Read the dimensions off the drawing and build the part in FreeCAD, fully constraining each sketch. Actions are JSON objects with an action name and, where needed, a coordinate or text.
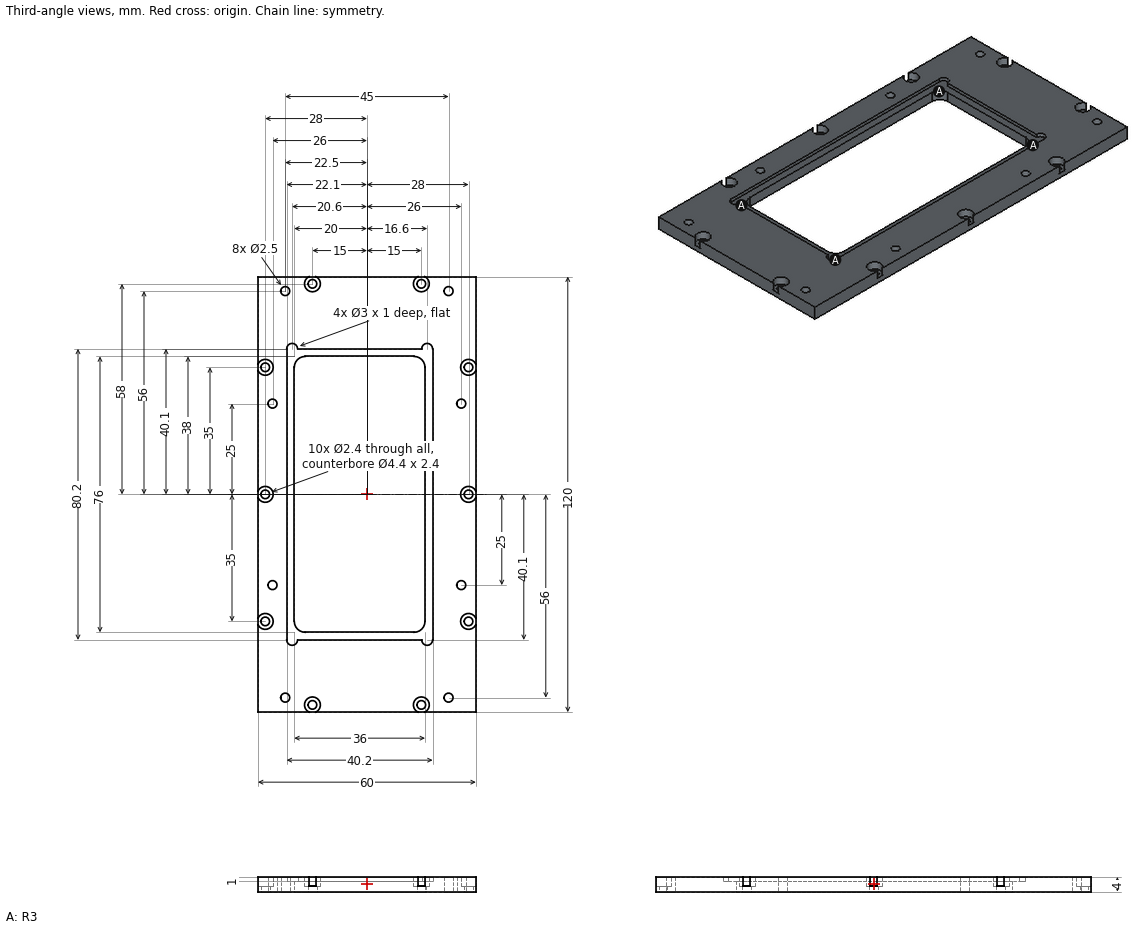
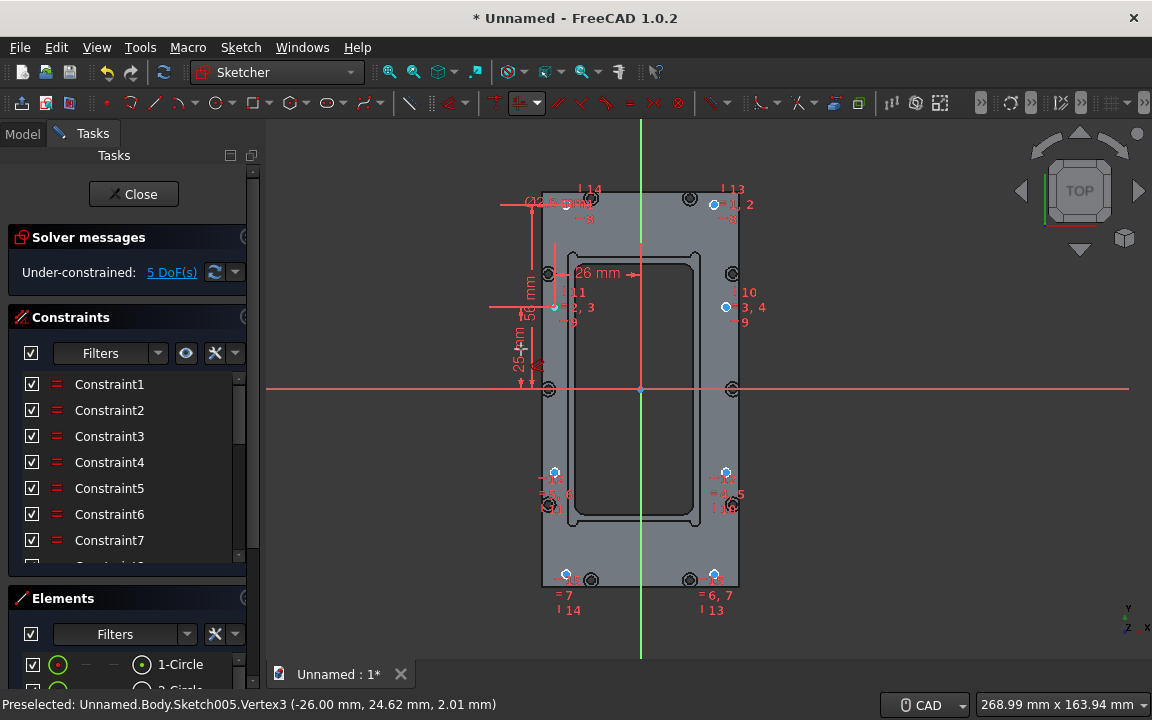
{"action": "left_click", "coordinate": [726, 307]}
{"action": "left_click", "coordinate": [683, 273]}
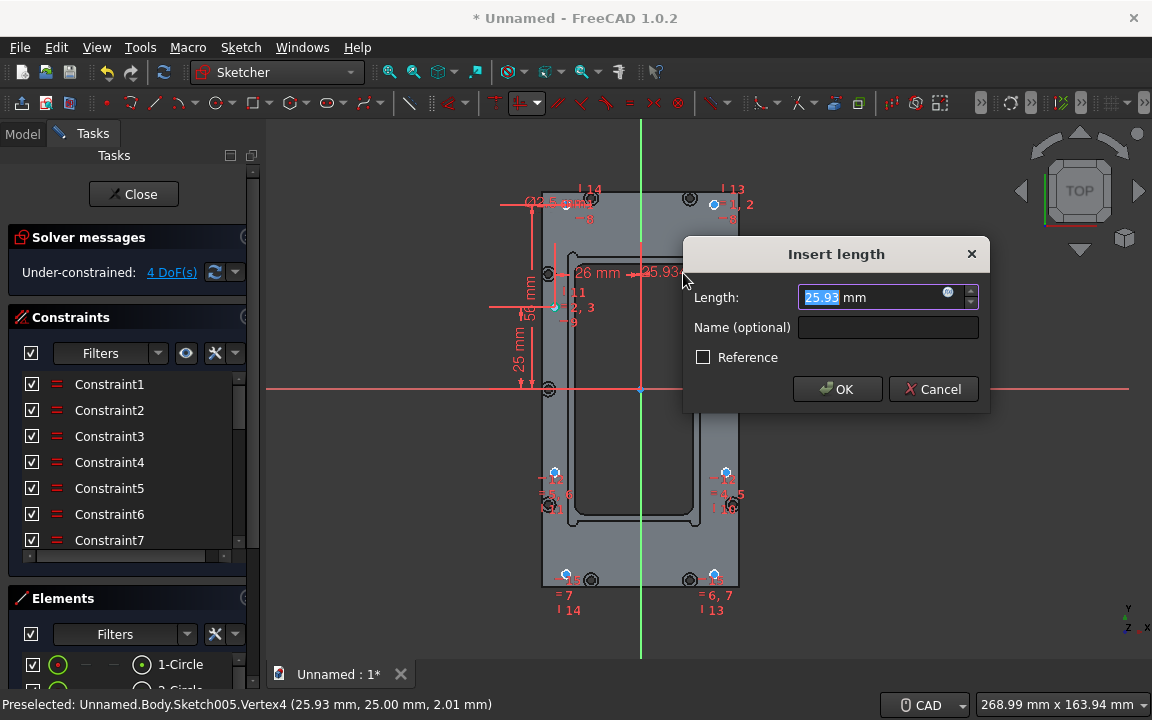
{"action": "type", "text": "26"}
{"action": "key", "text": "Return"}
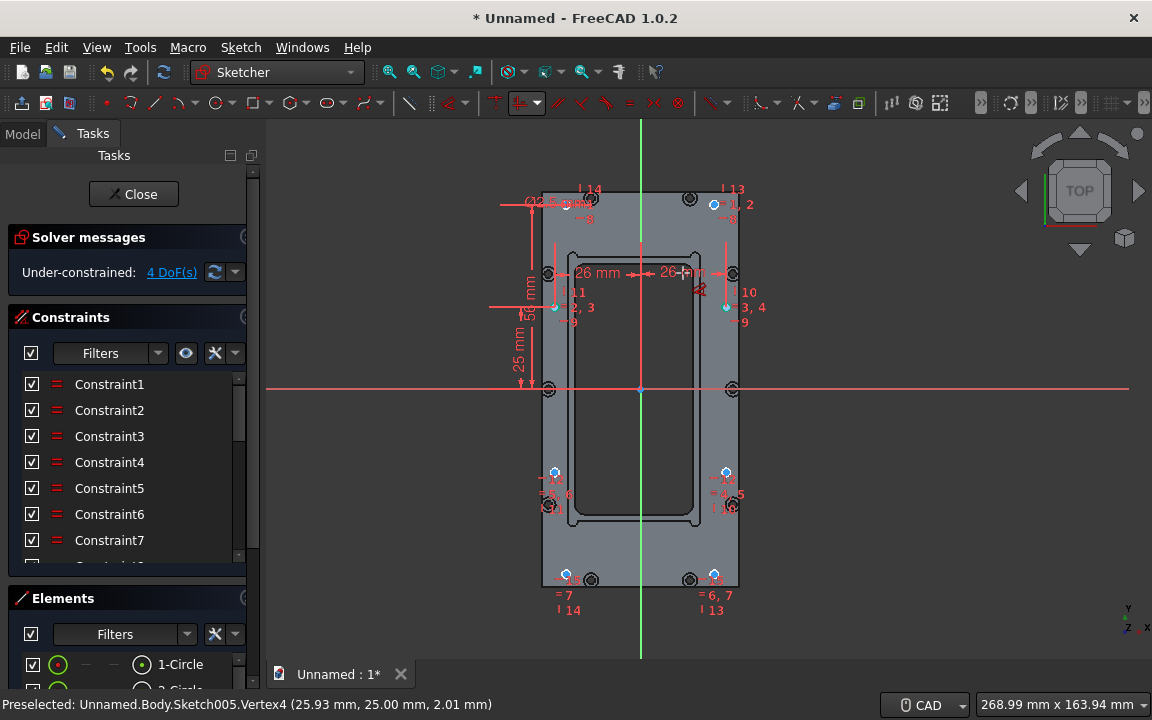
{"action": "left_click", "coordinate": [726, 472]}
{"action": "left_click", "coordinate": [760, 431]}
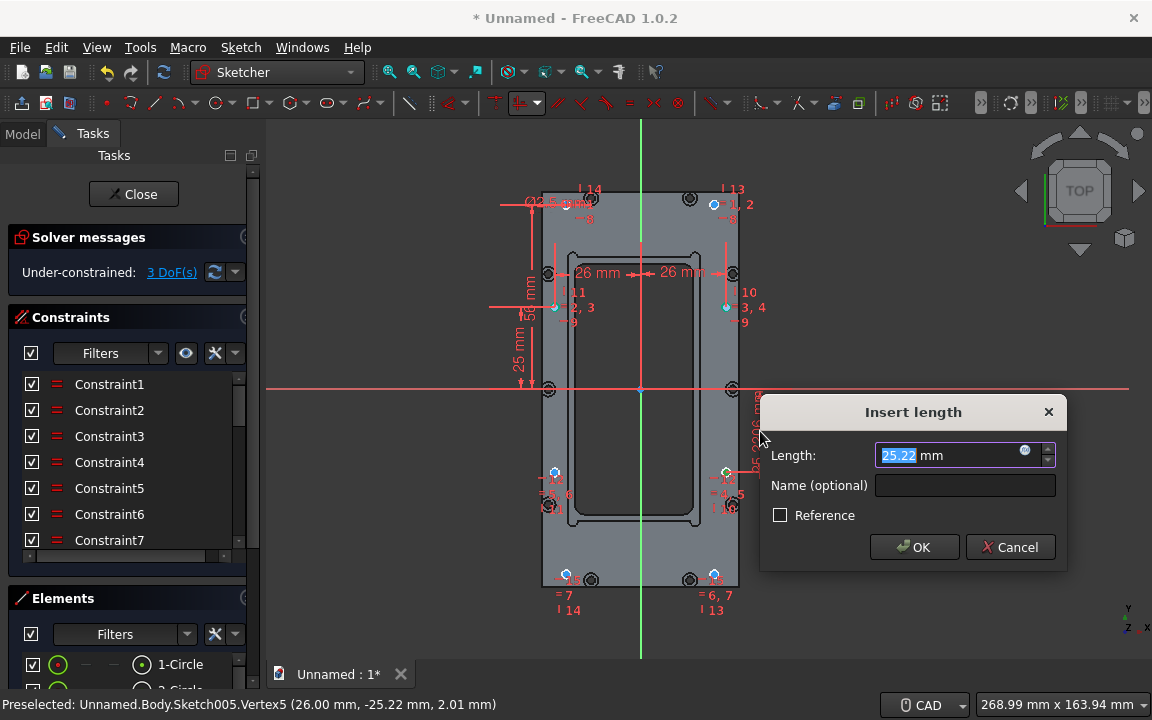
{"action": "type", "text": "25"}
{"action": "key", "text": "Return"}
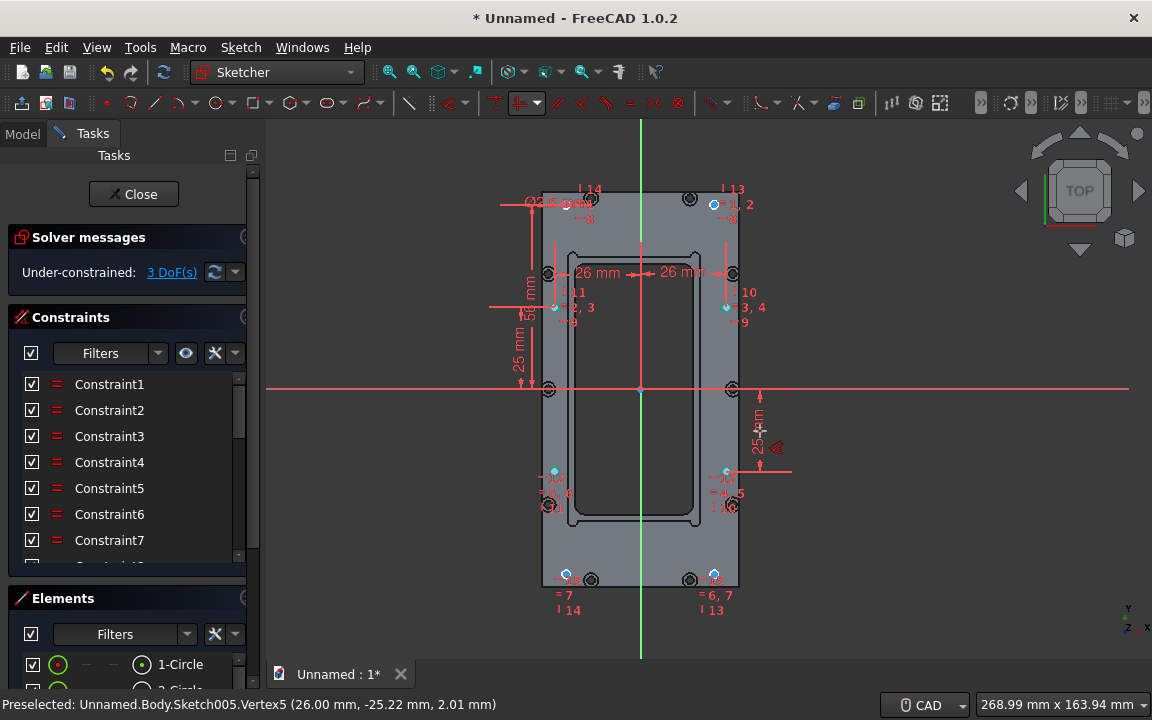
{"action": "left_click", "coordinate": [714, 574]}
{"action": "left_click", "coordinate": [748, 482]}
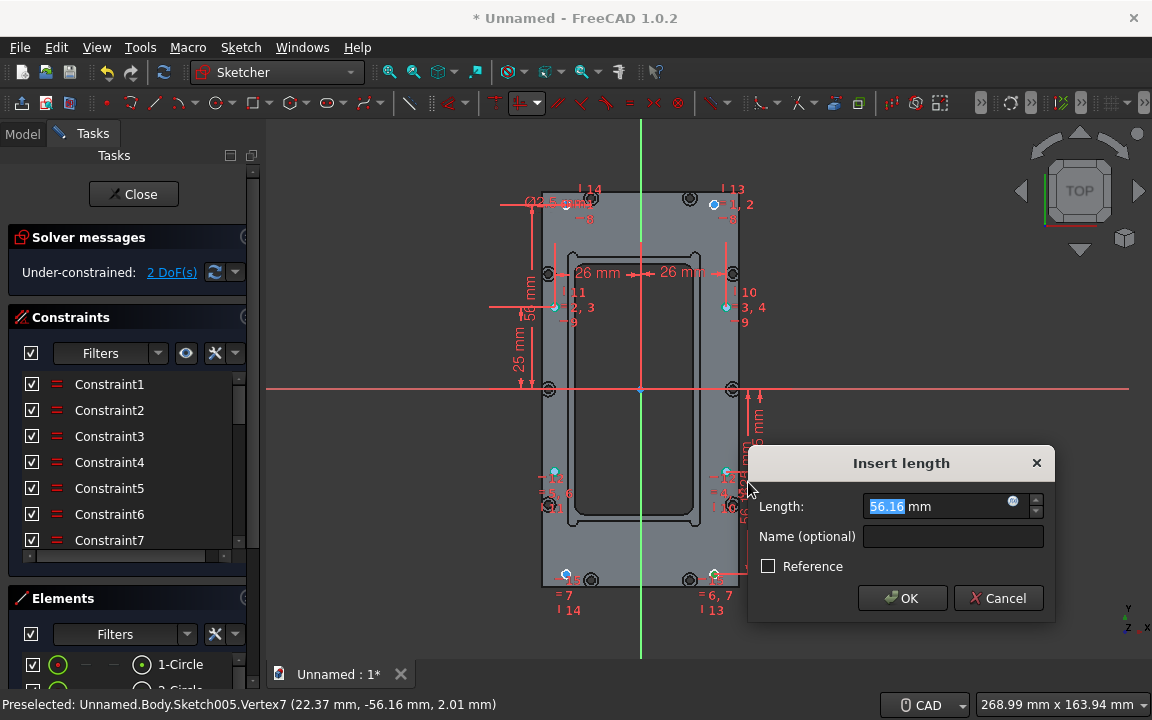
{"action": "type", "text": "56"}
{"action": "key", "text": "Return"}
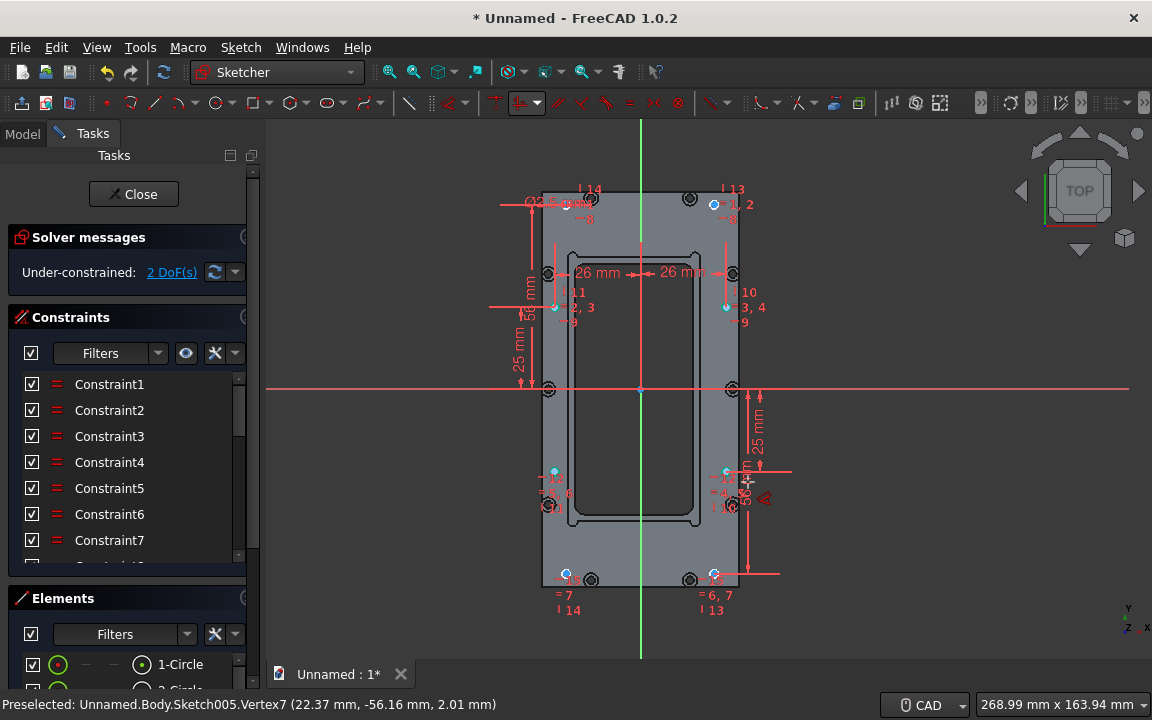
{"action": "left_click", "coordinate": [566, 205]}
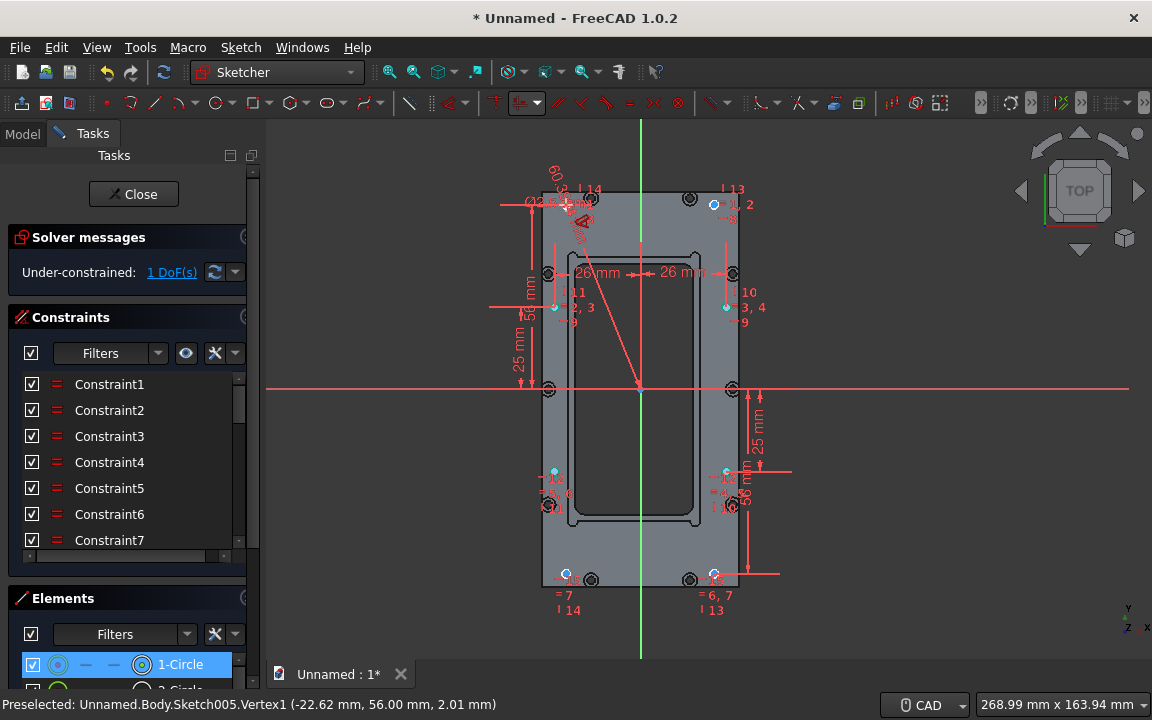
{"action": "left_click", "coordinate": [714, 205]}
{"action": "left_click", "coordinate": [606, 171]}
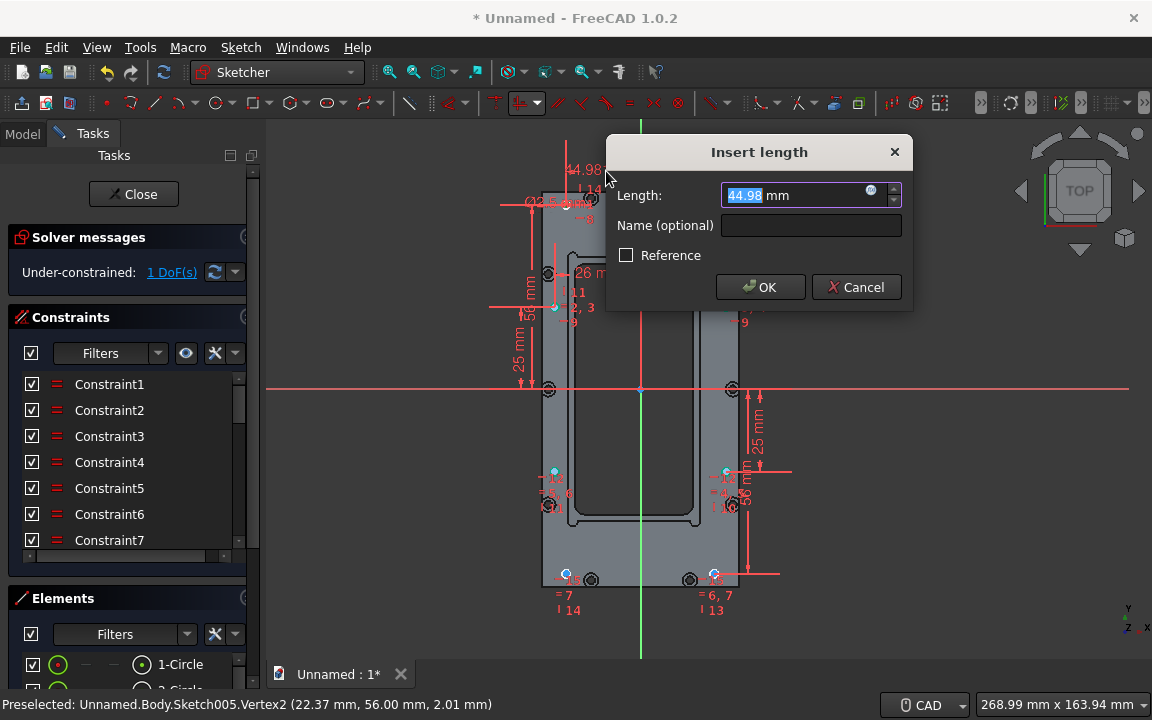
{"action": "type", "text": "45"}
{"action": "key", "text": "Return"}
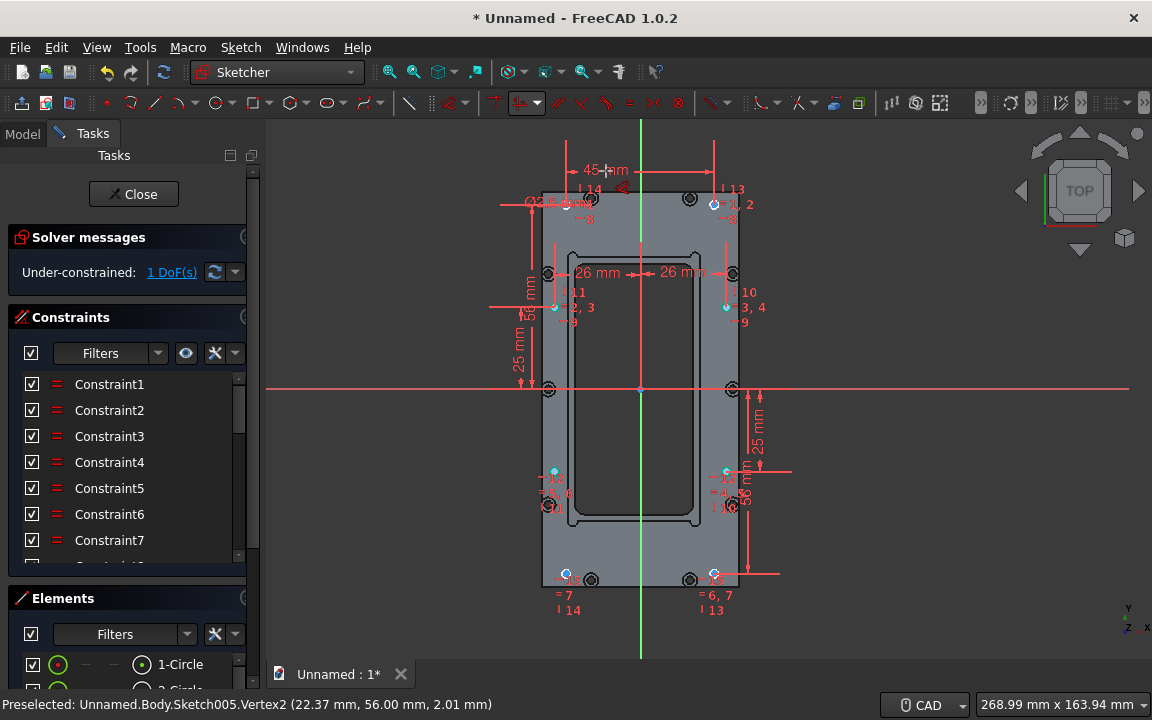
{"action": "left_click", "coordinate": [566, 205]}
{"action": "left_click", "coordinate": [603, 423]}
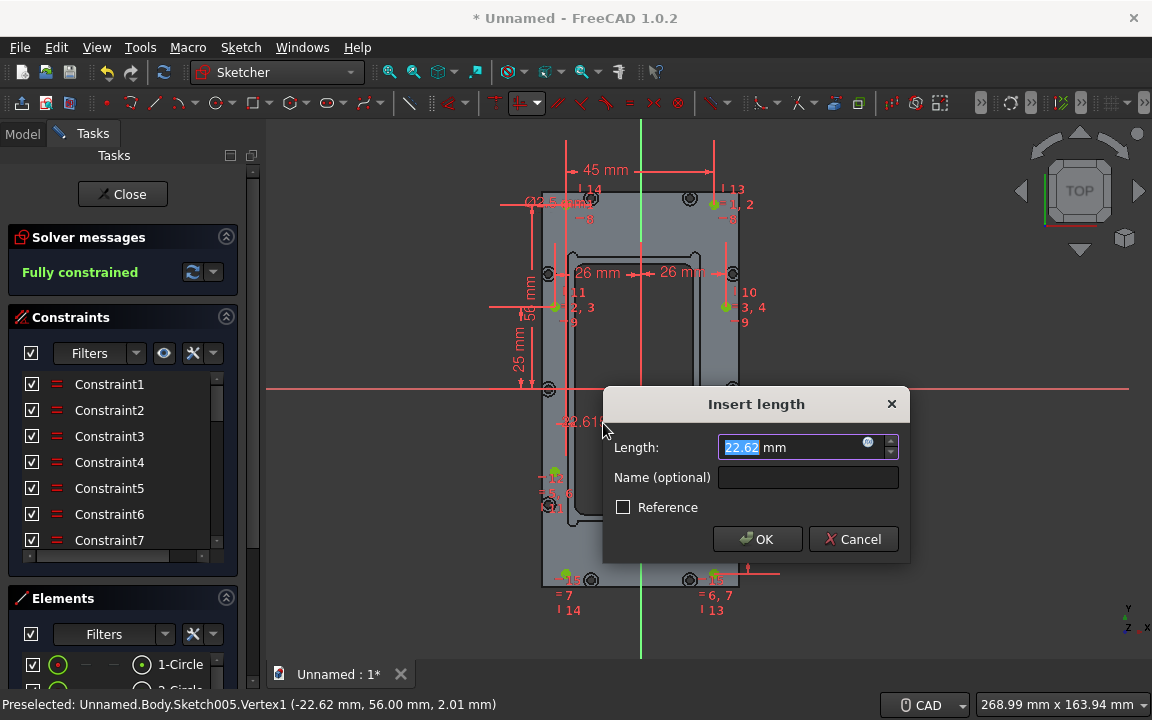
{"action": "type", "text": "22.5"}
{"action": "key", "text": "Return"}
{"action": "key", "text": "Escape"}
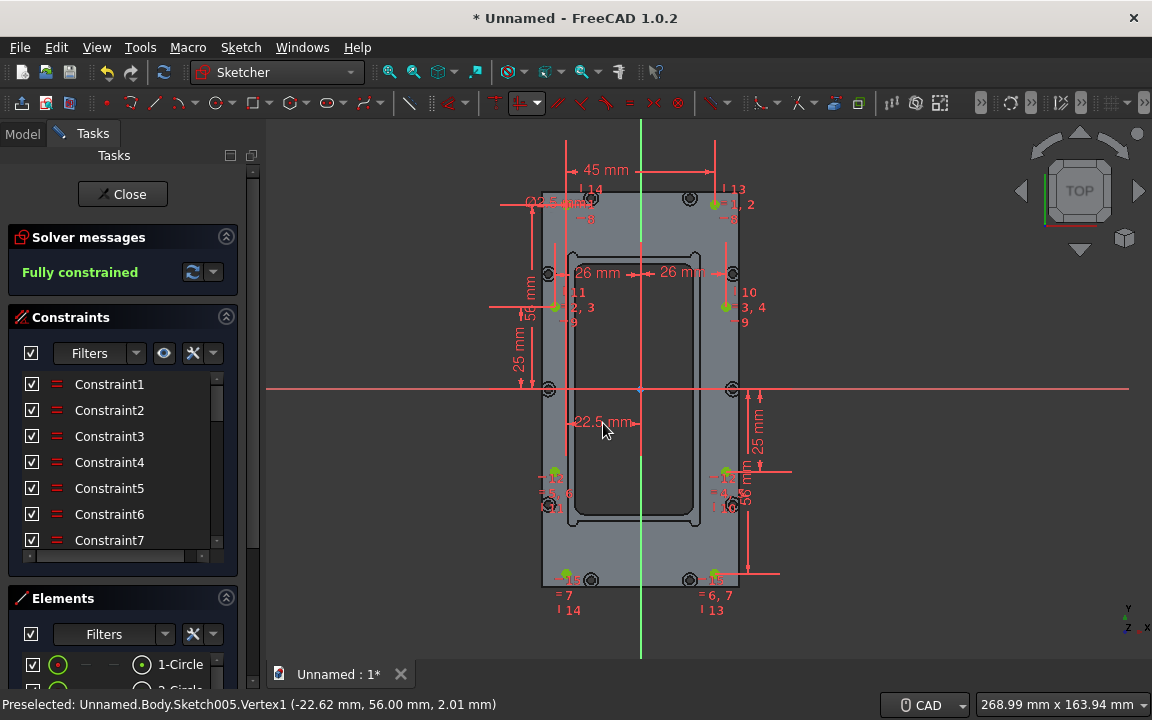
{"action": "left_click", "coordinate": [123, 194]}